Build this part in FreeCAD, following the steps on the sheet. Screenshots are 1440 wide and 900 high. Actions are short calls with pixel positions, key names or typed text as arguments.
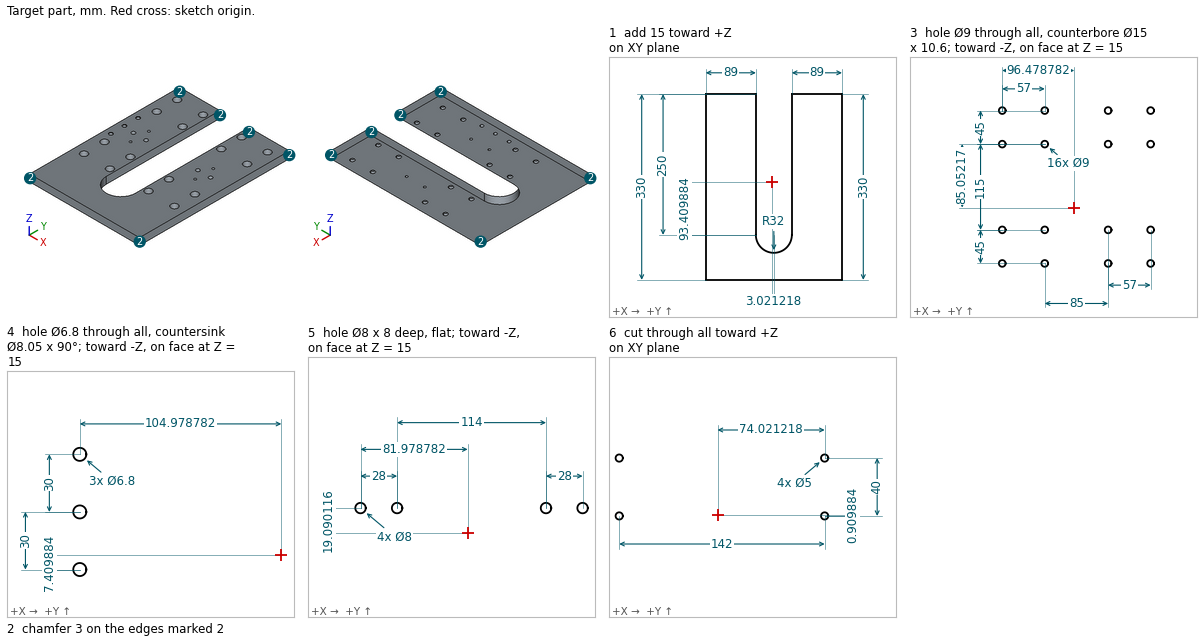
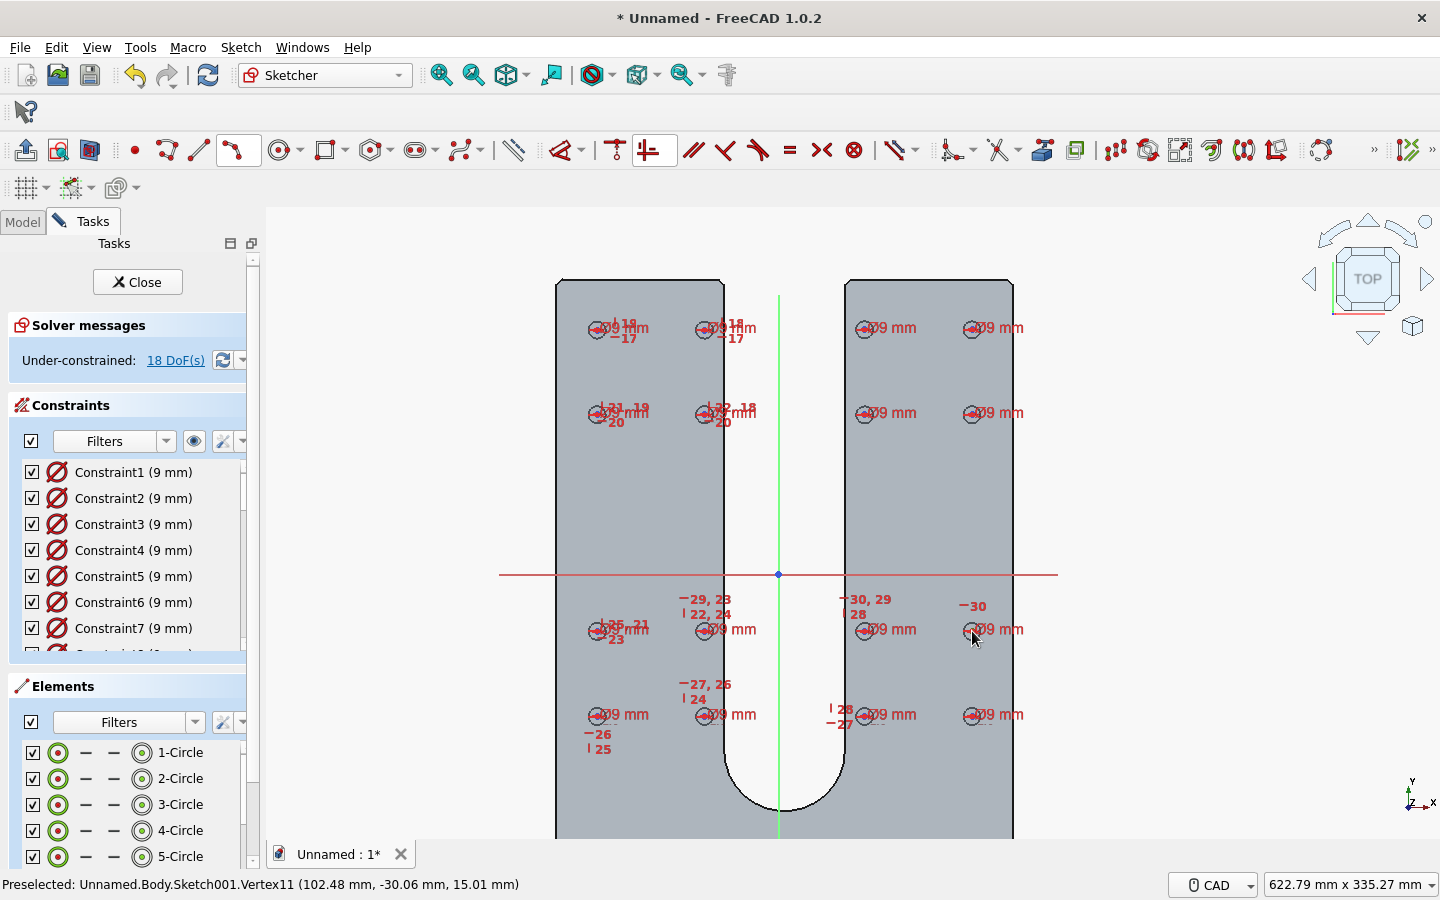
click(972, 717)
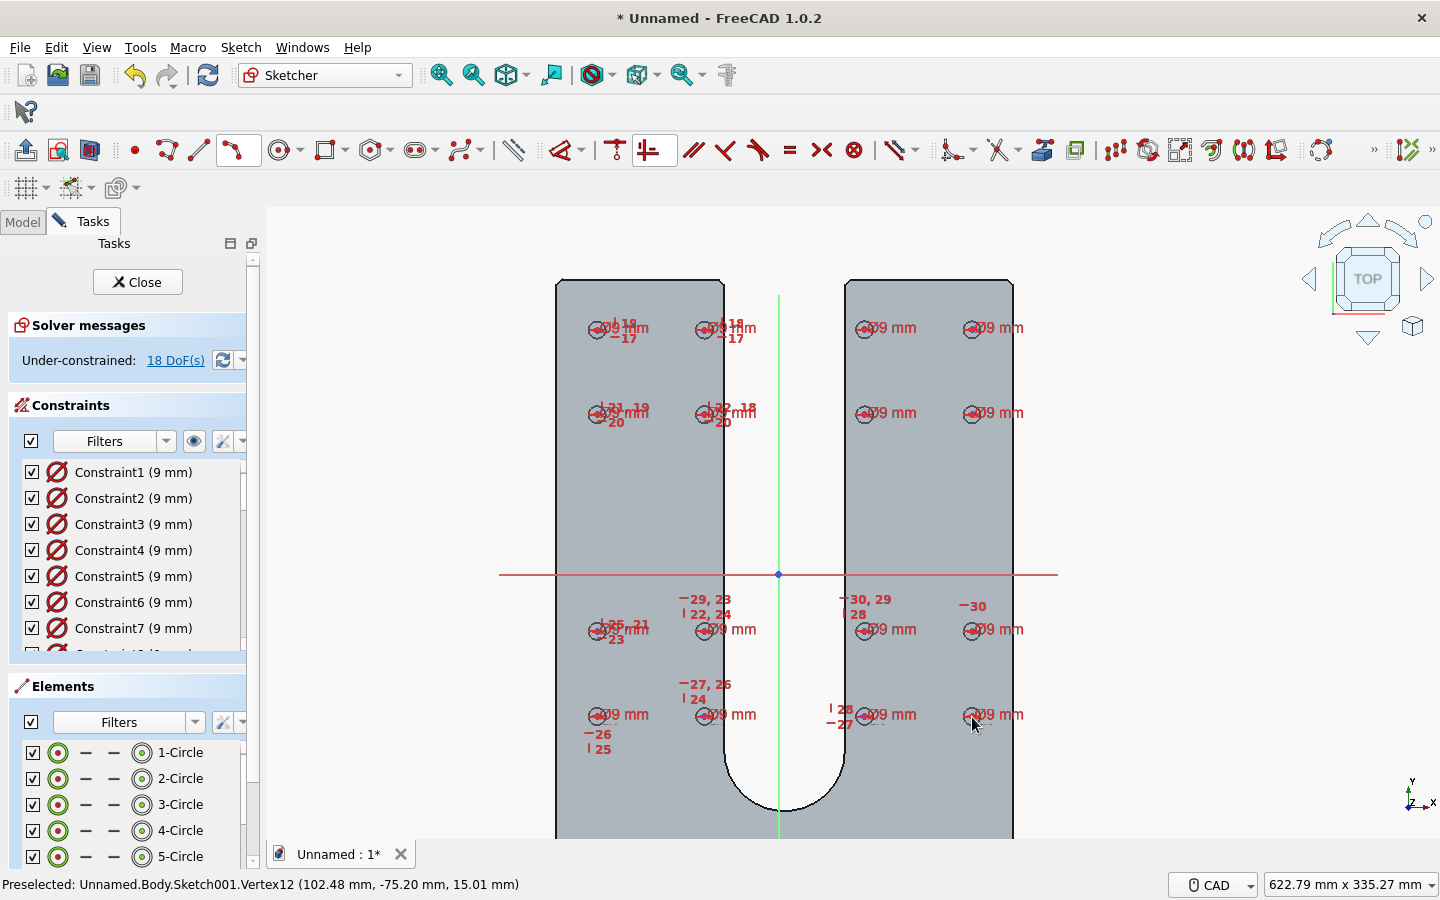
key(v)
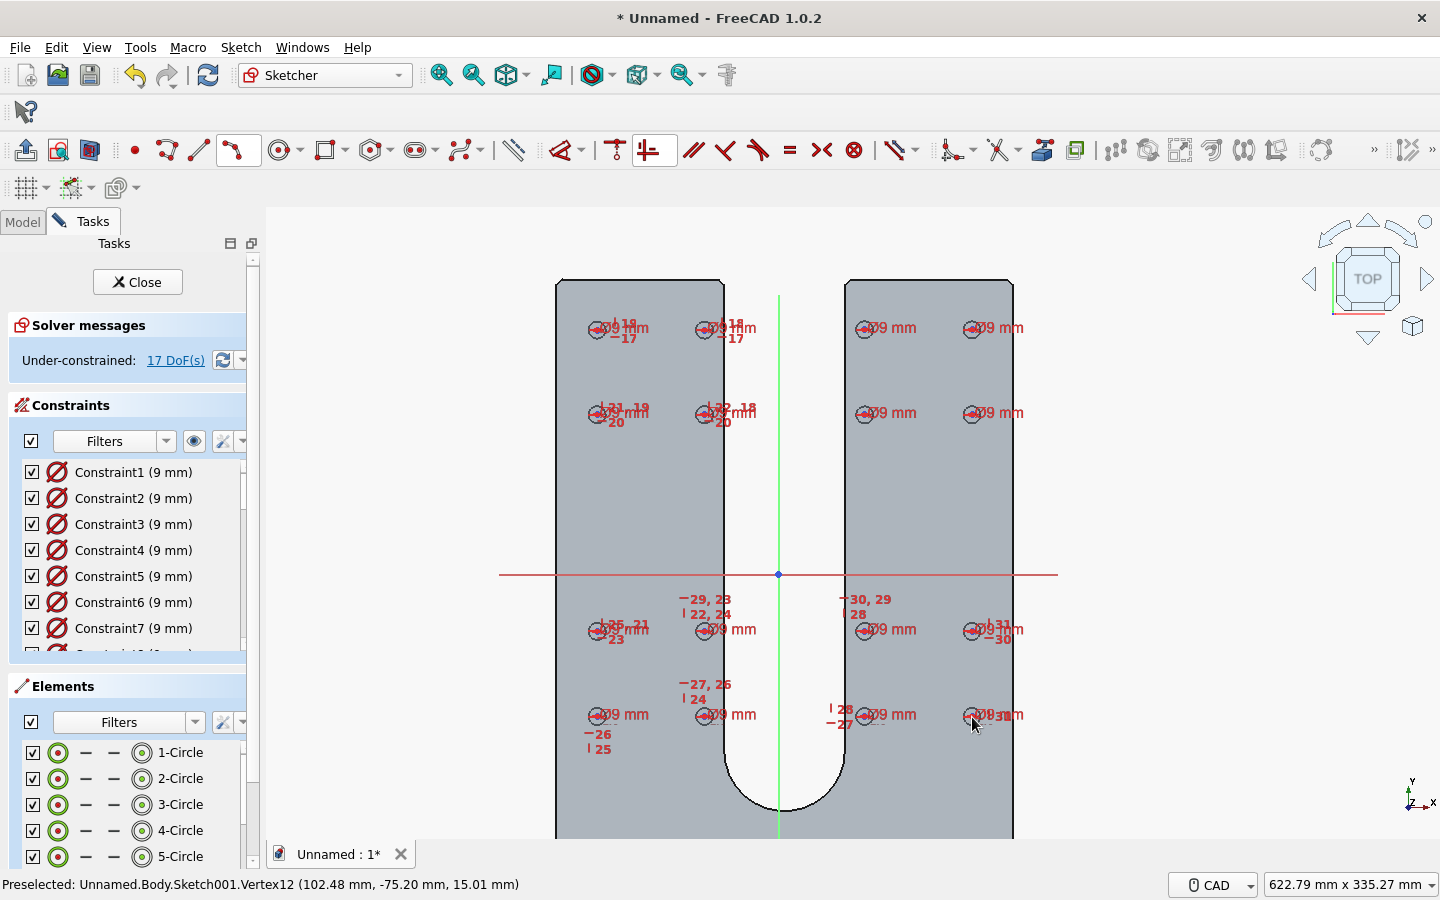
click(865, 717)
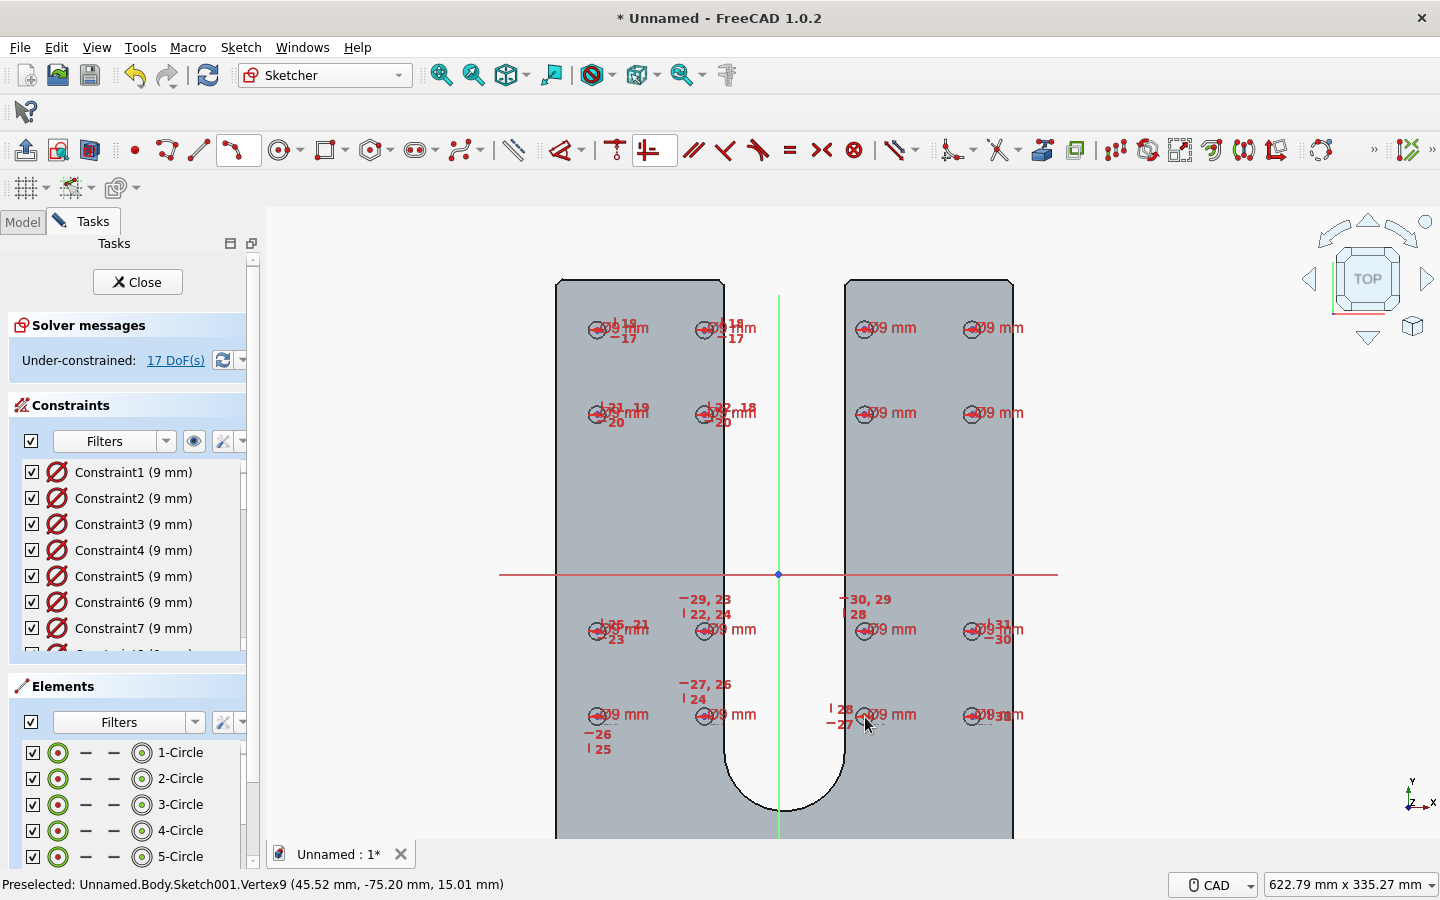
click(972, 717)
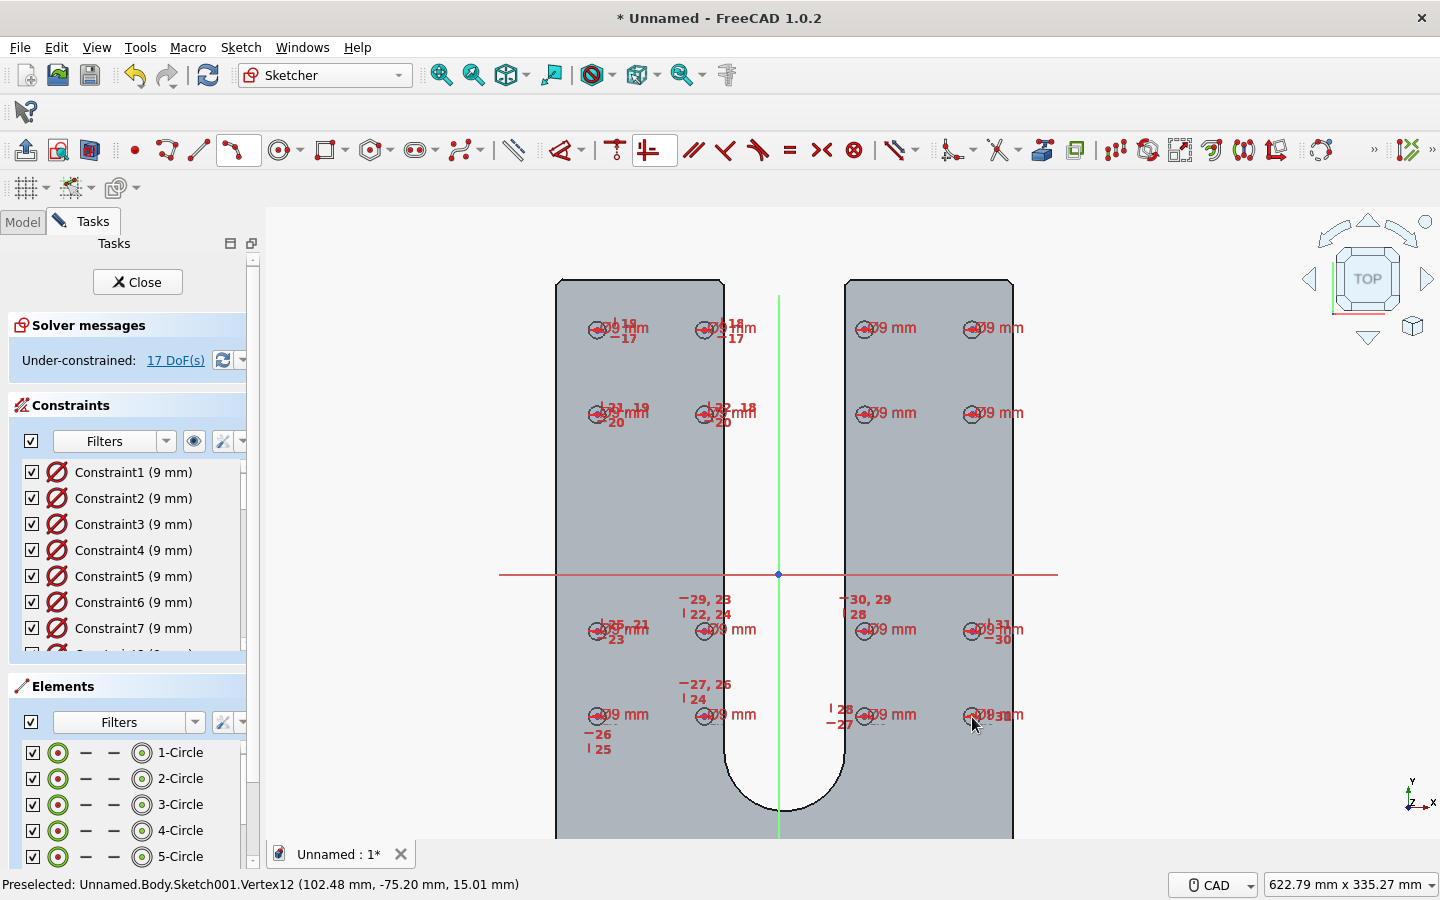
key(h)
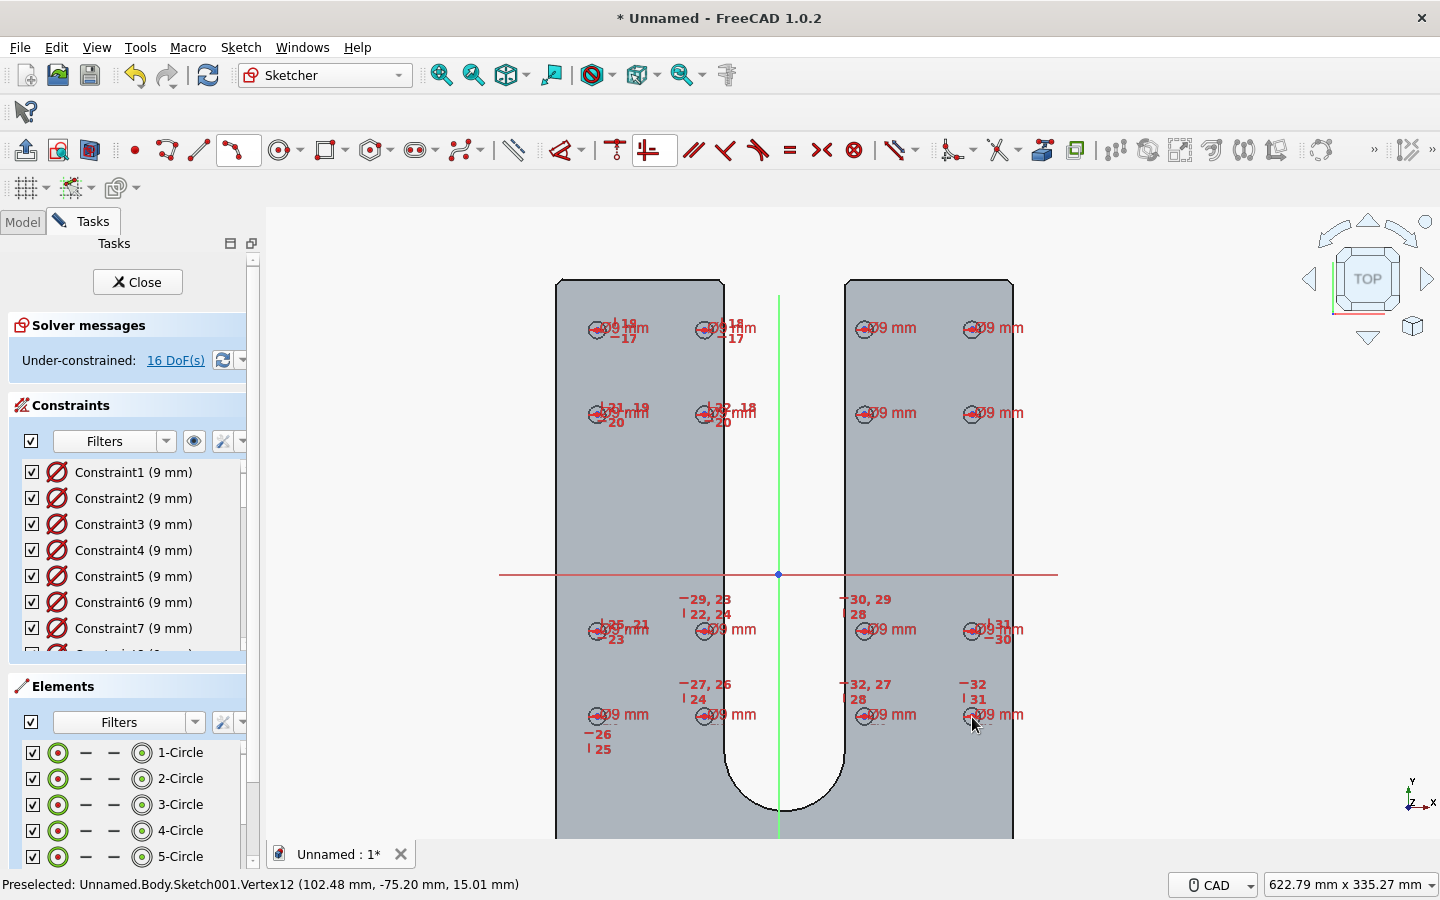
click(865, 631)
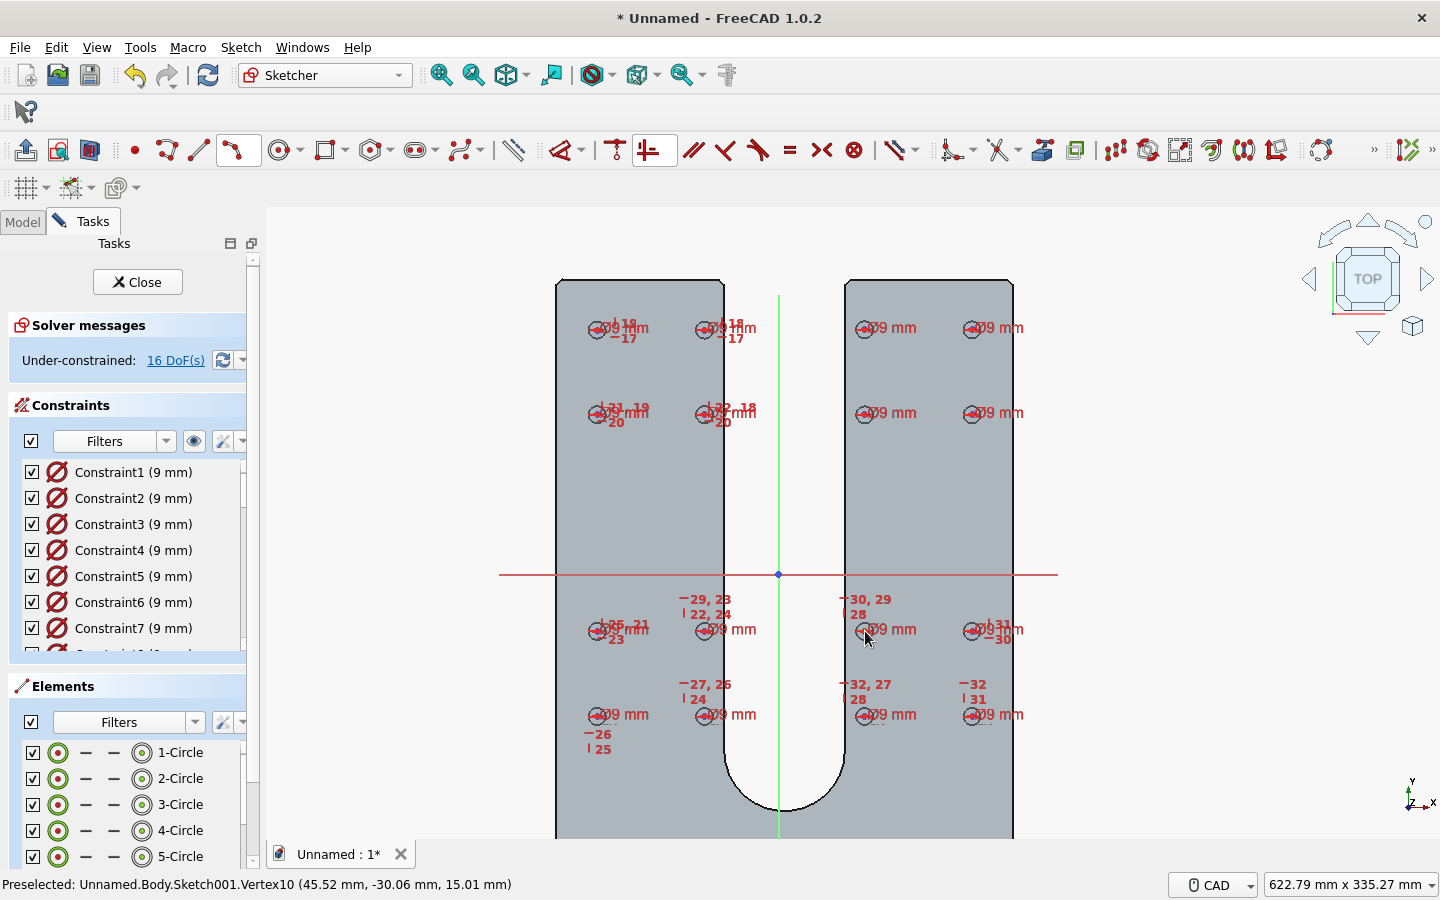
click(865, 415)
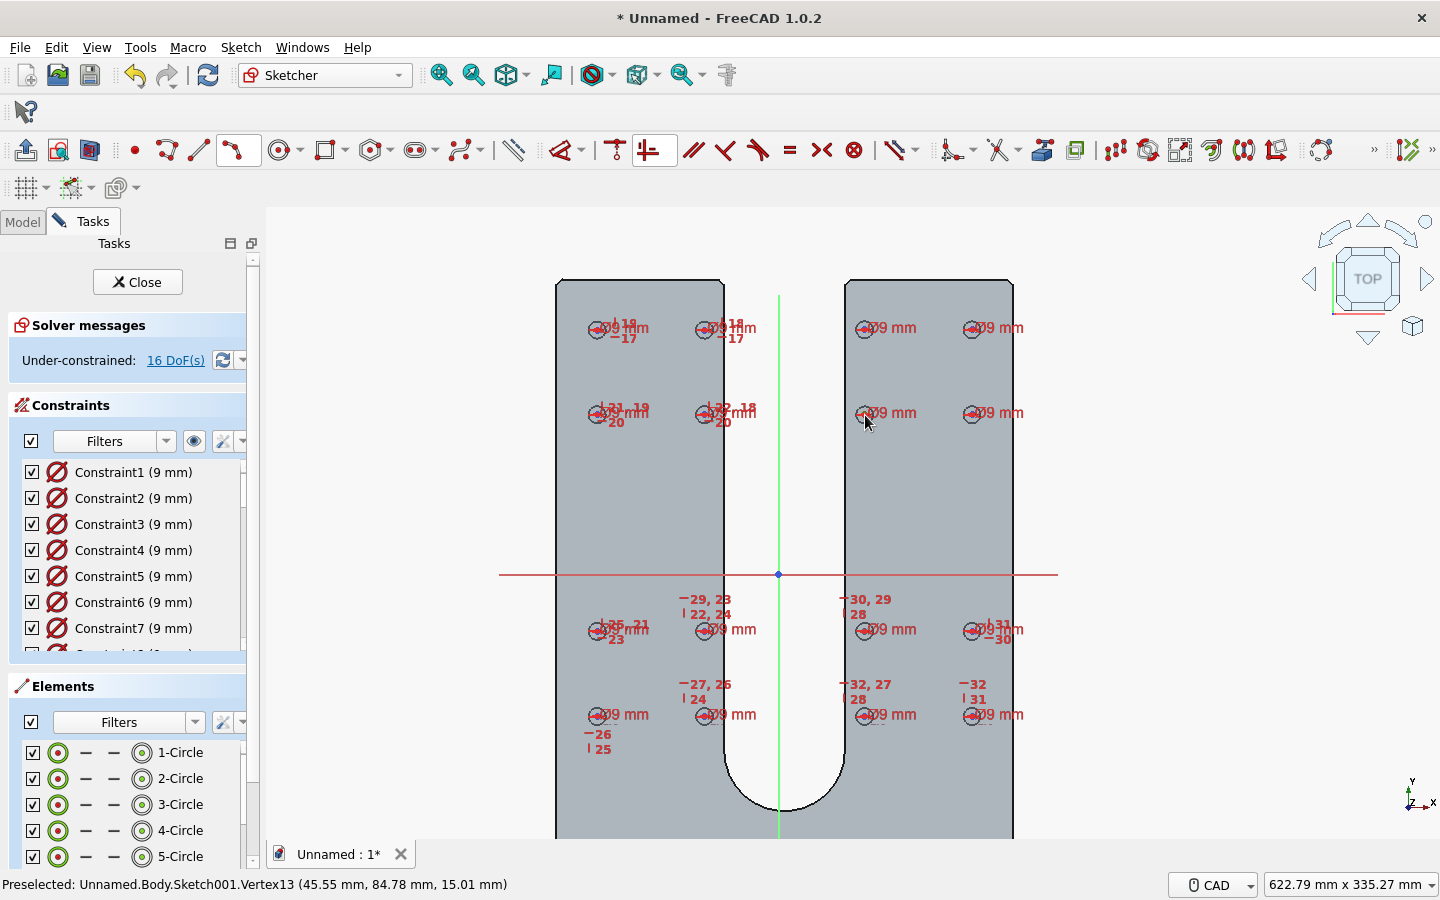
key(v)